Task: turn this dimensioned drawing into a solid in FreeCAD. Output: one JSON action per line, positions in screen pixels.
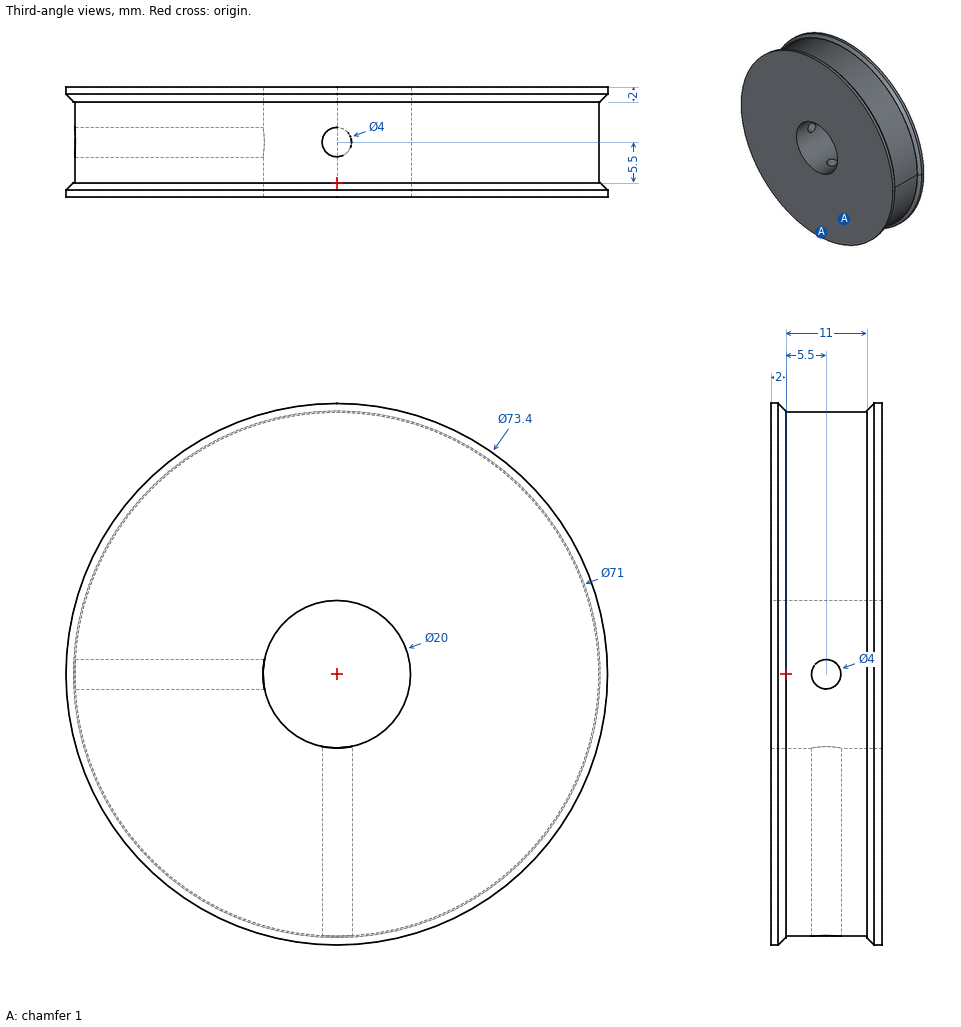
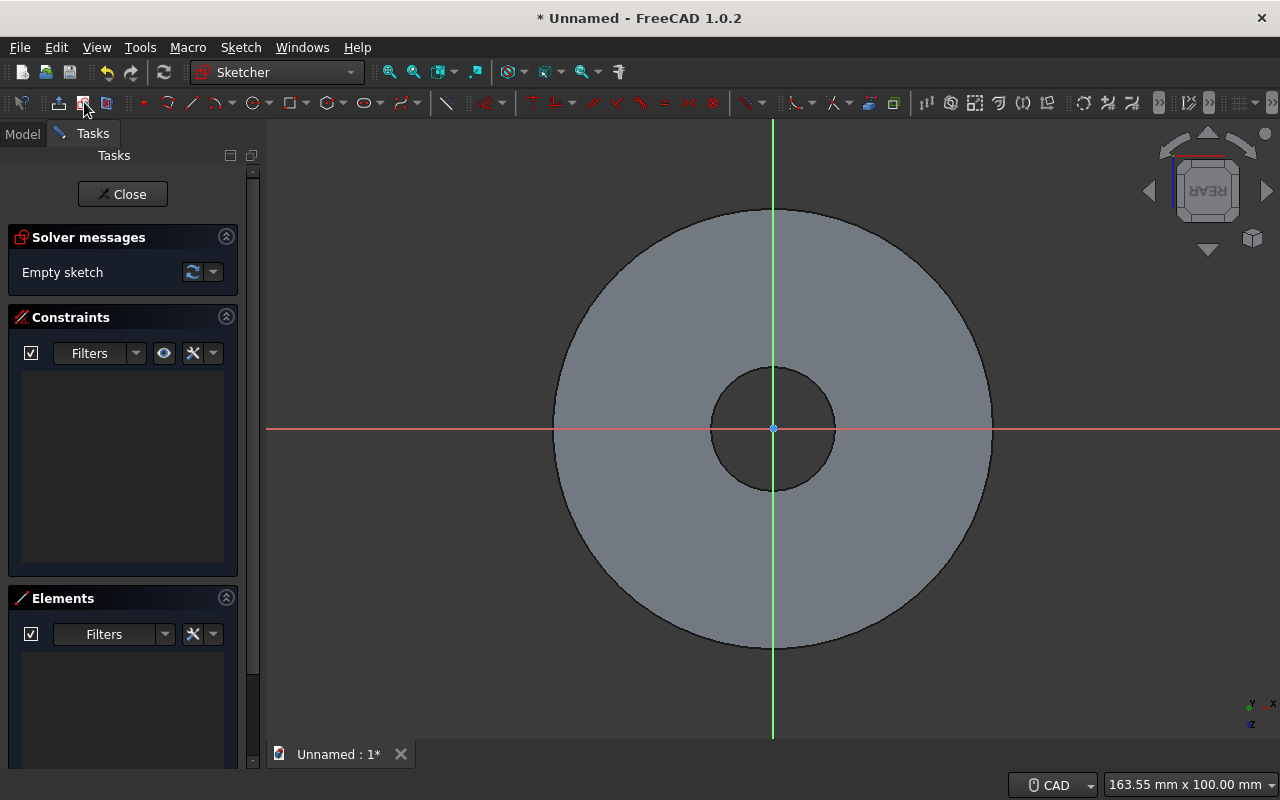
{"action": "left_click", "coordinate": [254, 104]}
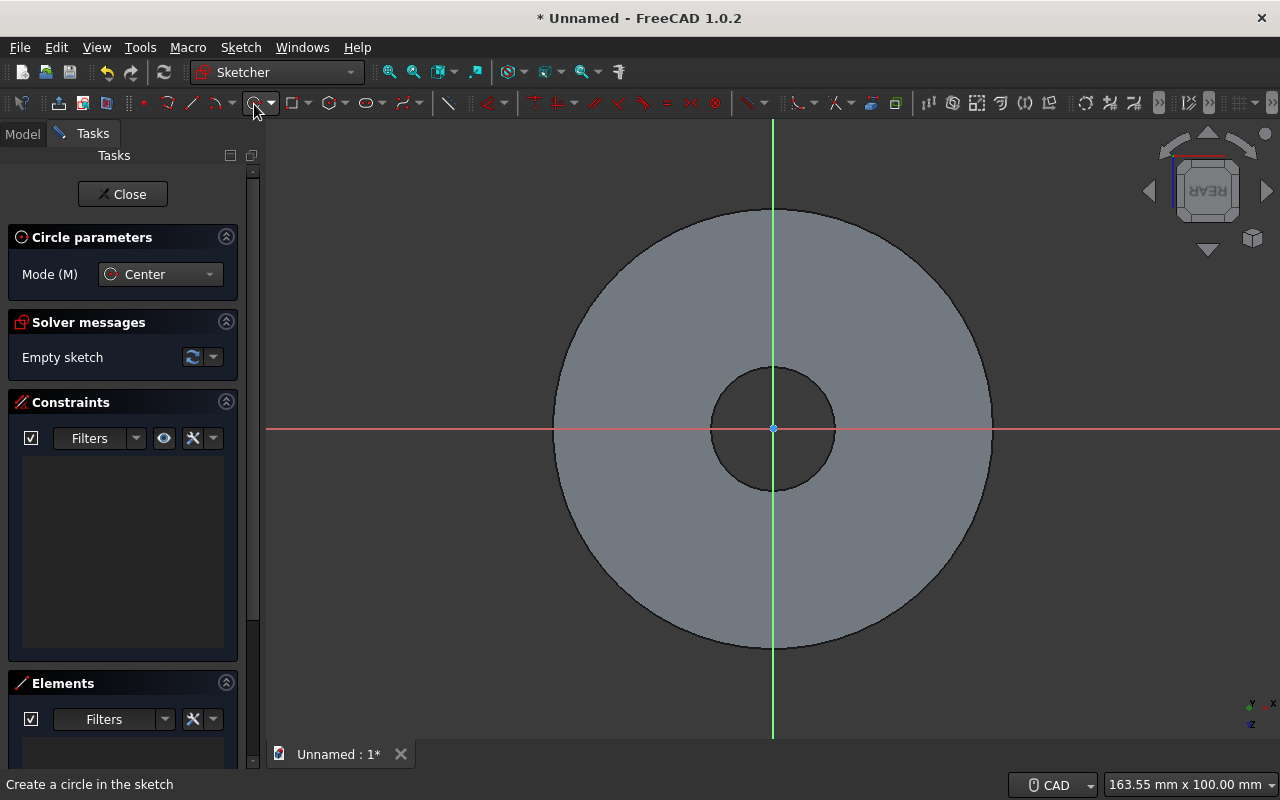
{"action": "left_click", "coordinate": [773, 429]}
{"action": "left_click", "coordinate": [934, 268]}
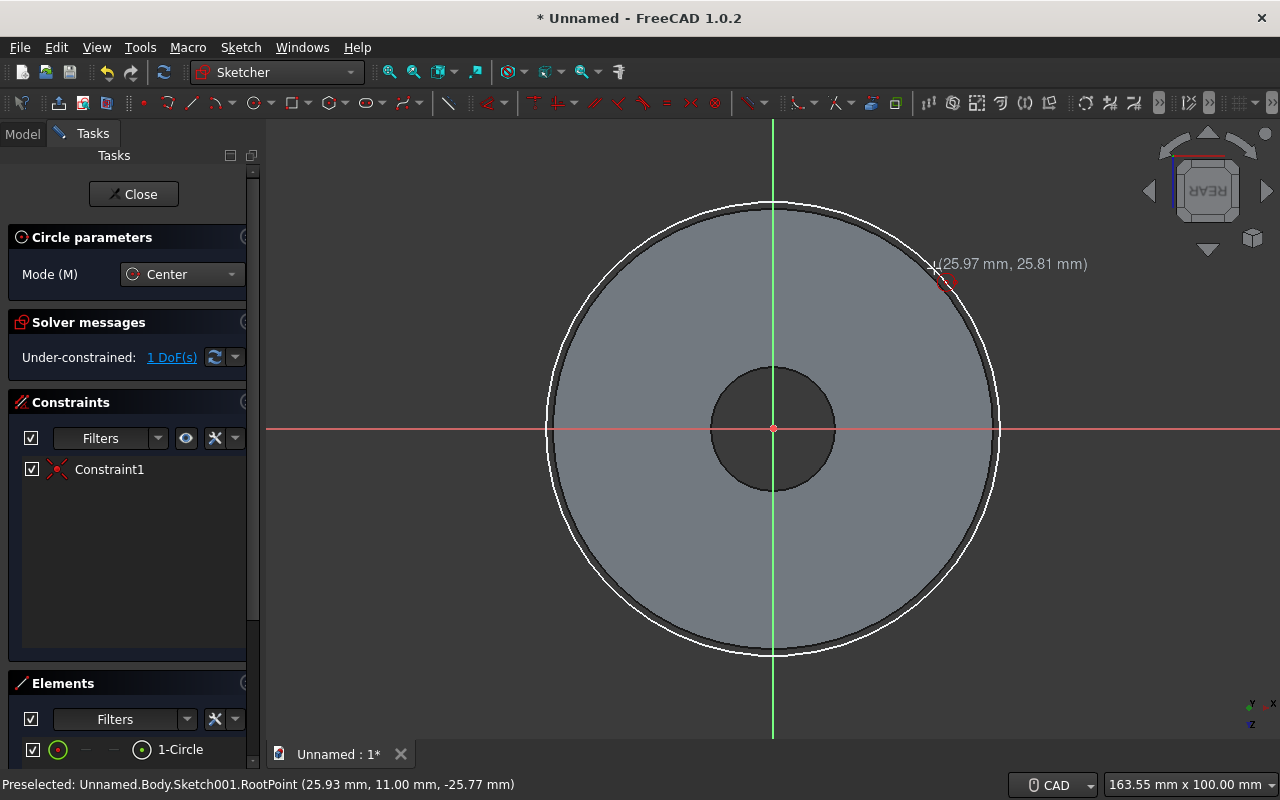
{"action": "left_click", "coordinate": [773, 429]}
{"action": "left_click", "coordinate": [817, 385]}
{"action": "key", "text": "Escape"}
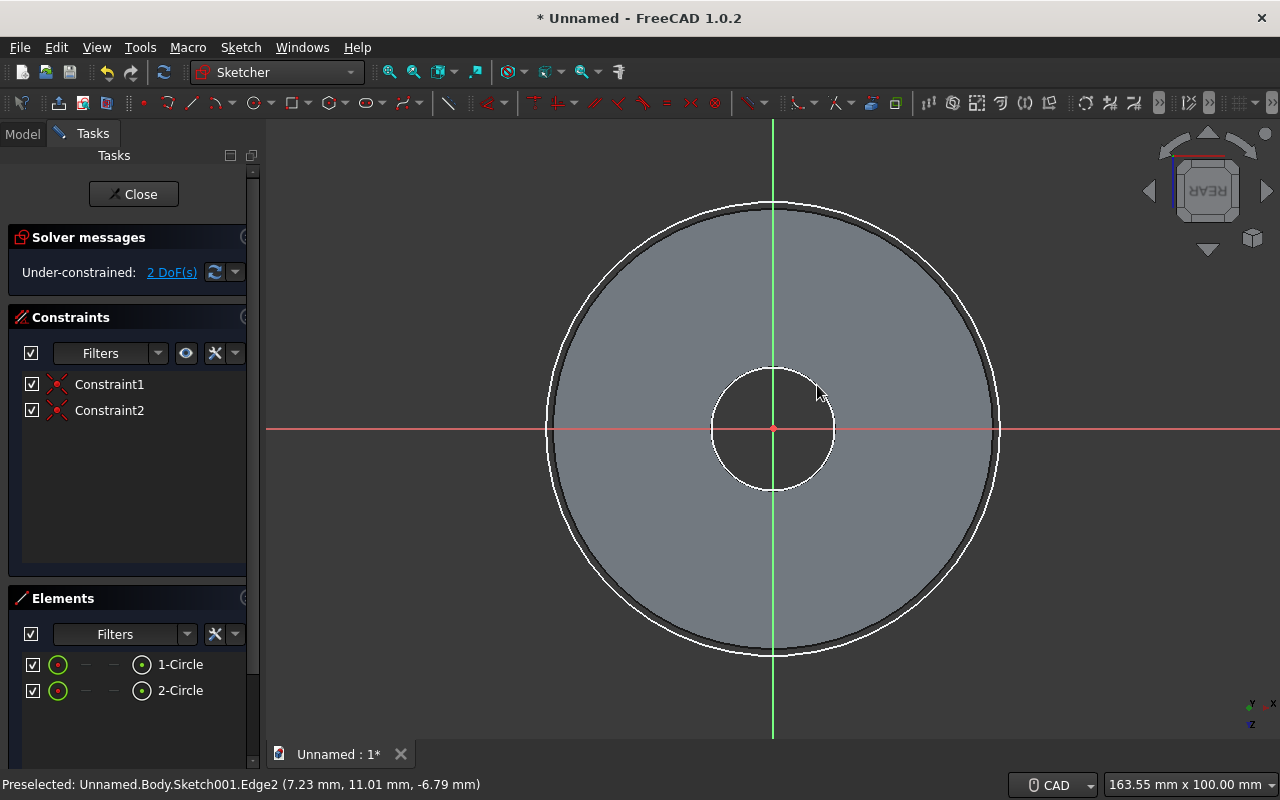
{"action": "left_click", "coordinate": [488, 104]}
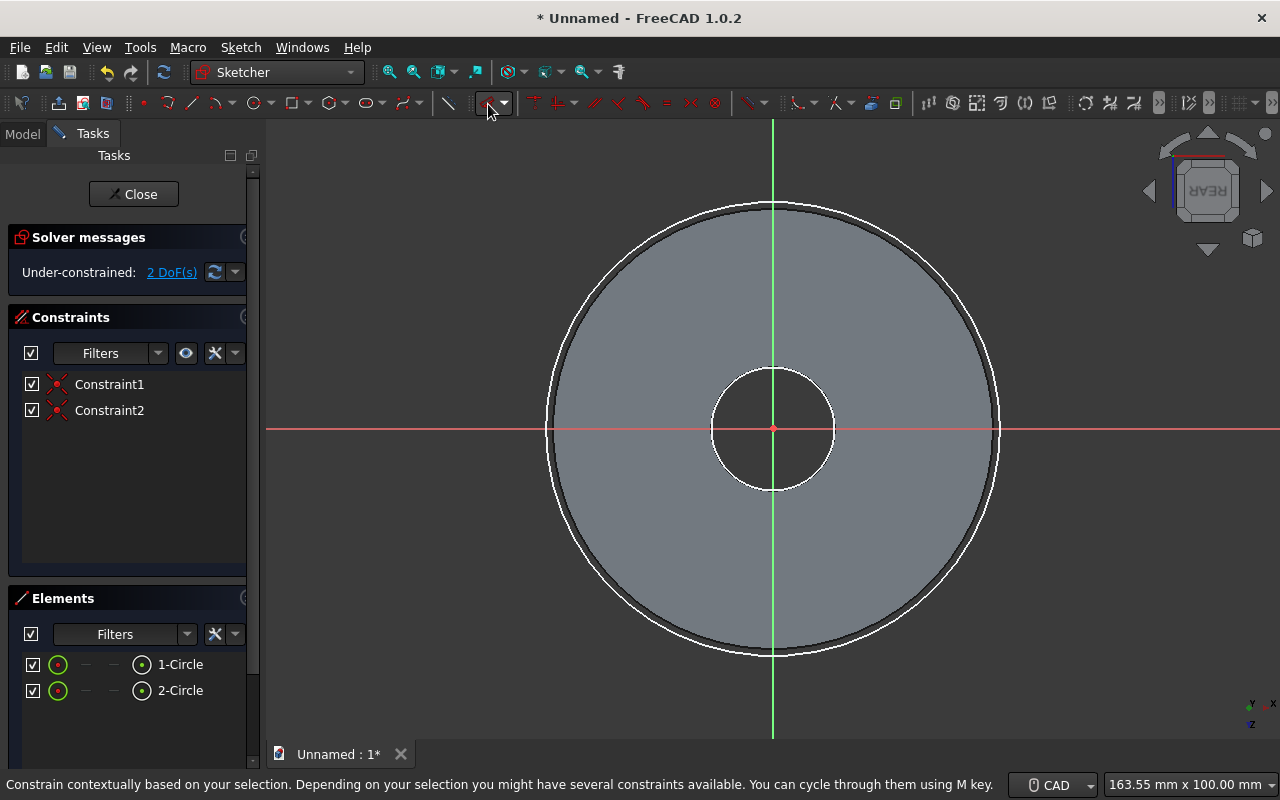
{"action": "left_click", "coordinate": [933, 268]}
{"action": "left_click", "coordinate": [956, 245]}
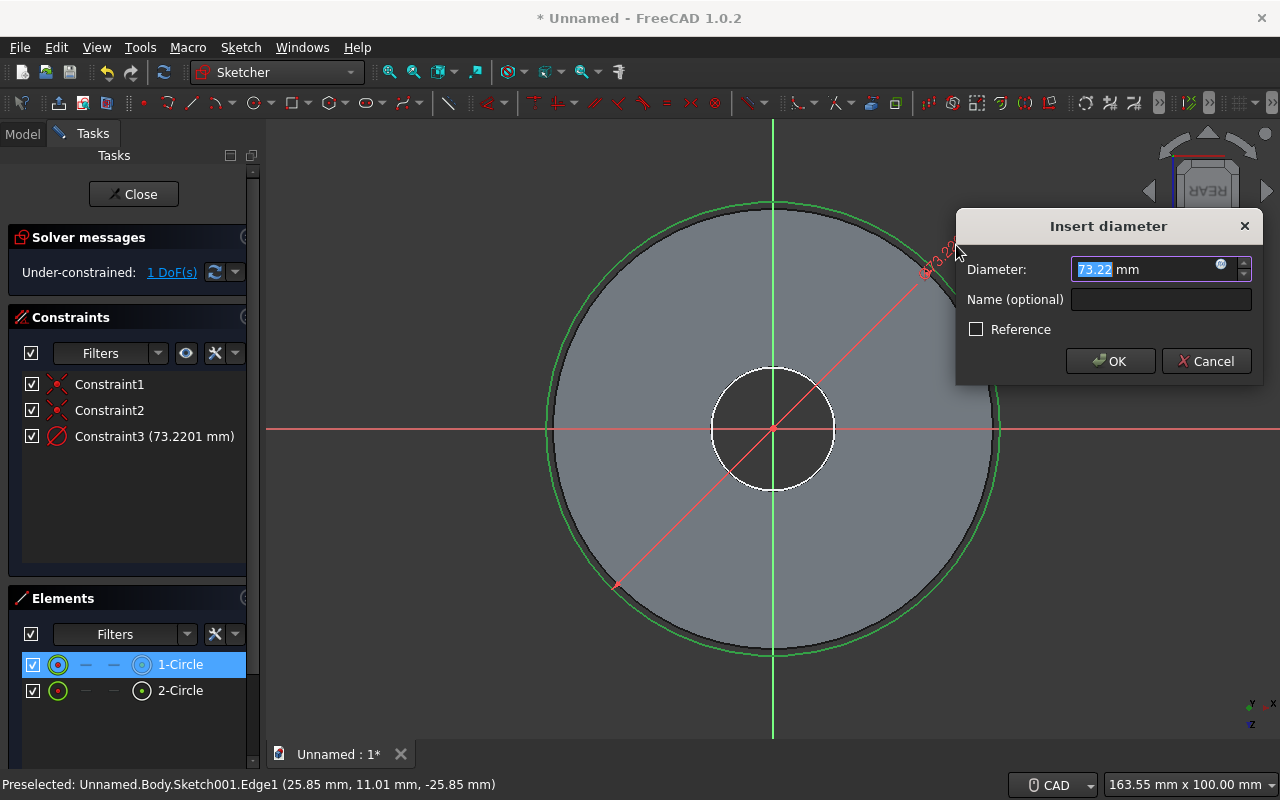
{"action": "type", "text": "73.4"}
{"action": "key", "text": "Return"}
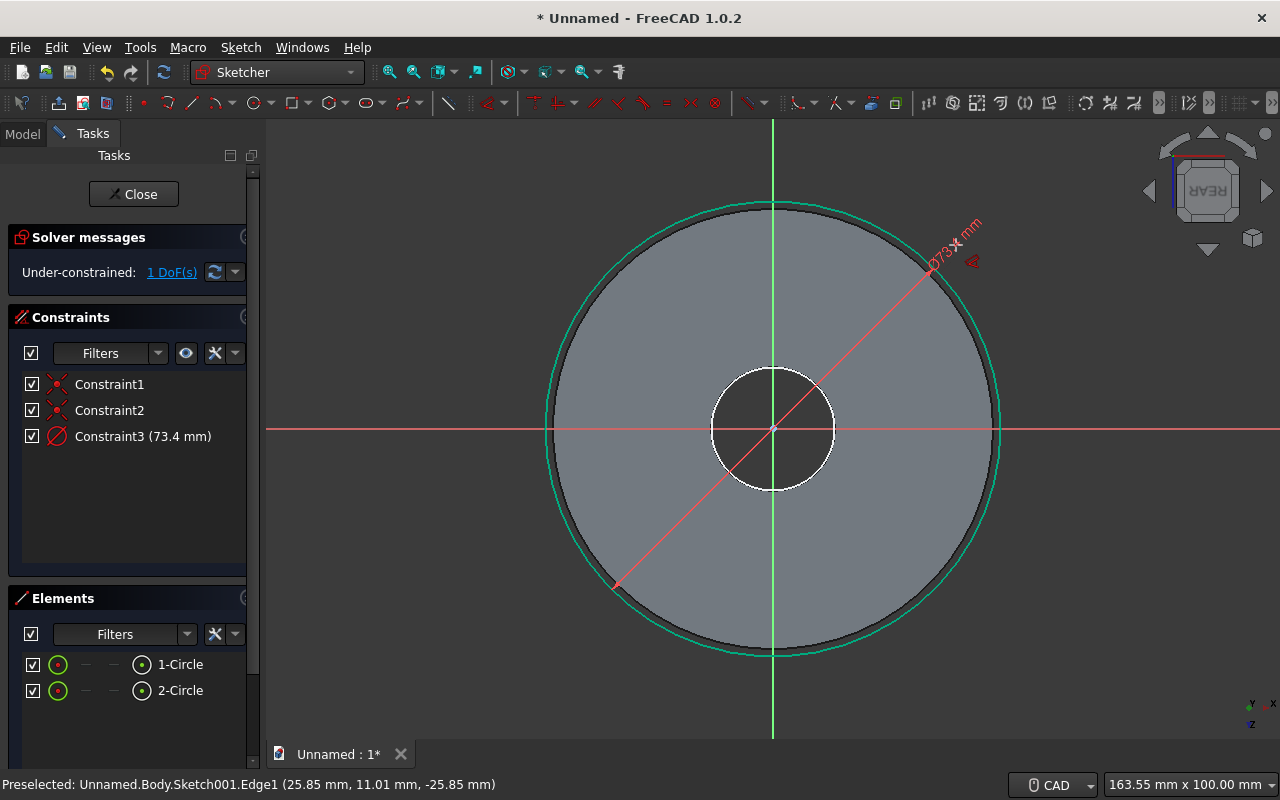
{"action": "left_click", "coordinate": [816, 385]}
{"action": "left_click", "coordinate": [838, 362]}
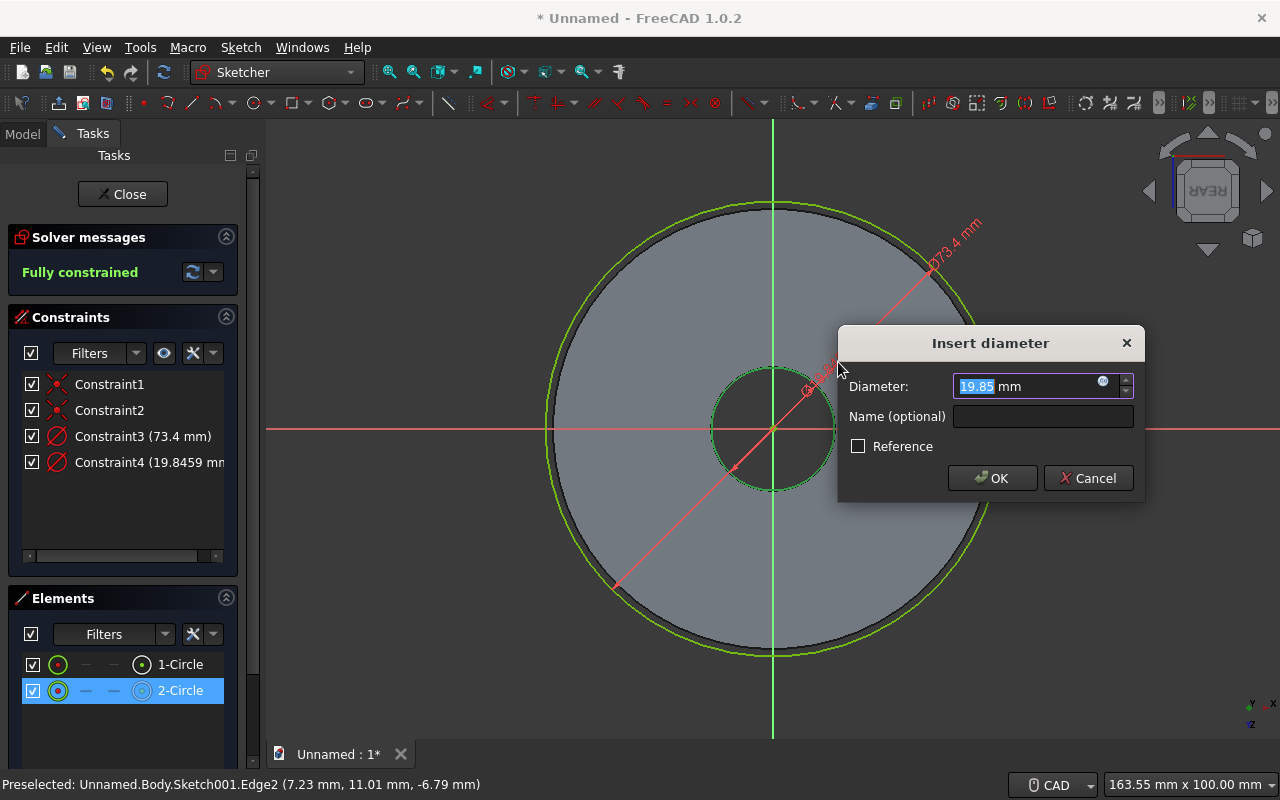
{"action": "type", "text": "20"}
{"action": "key", "text": "Return"}
{"action": "key", "text": "Escape"}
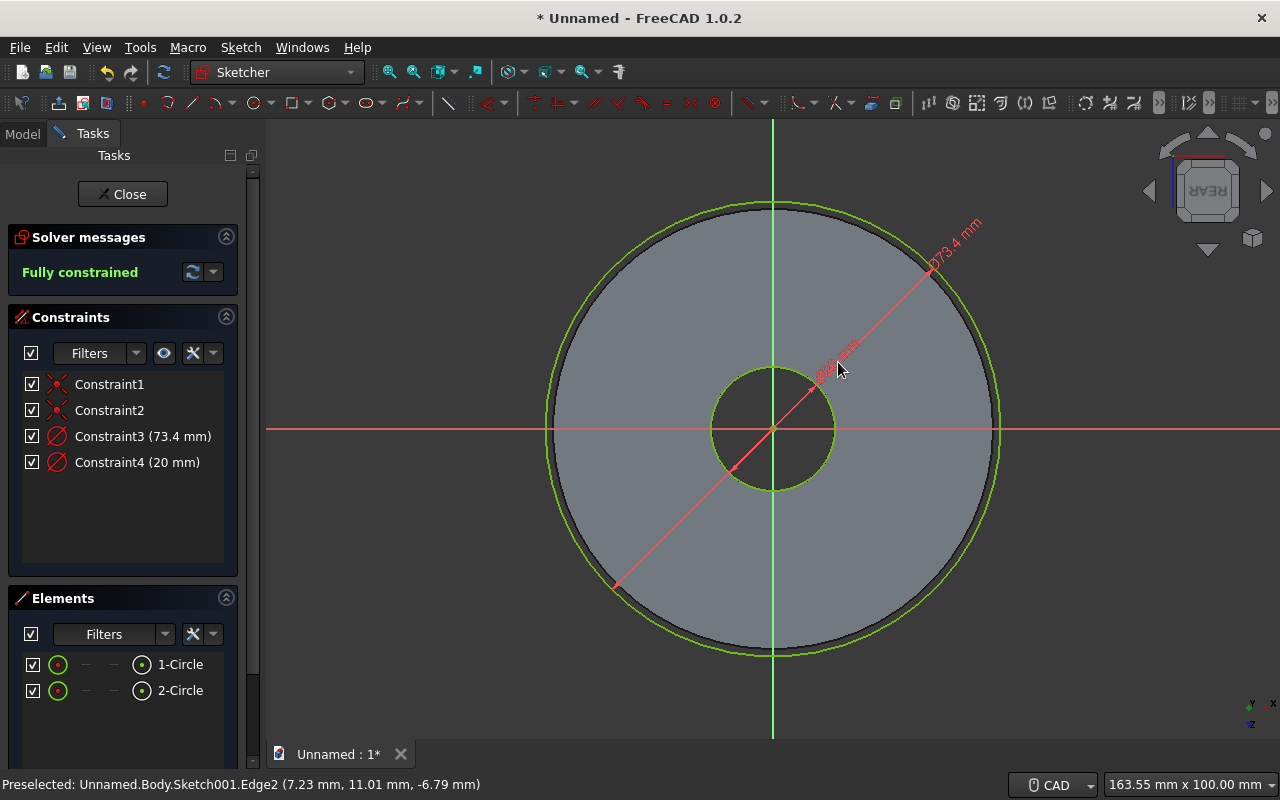
{"action": "left_click", "coordinate": [123, 194]}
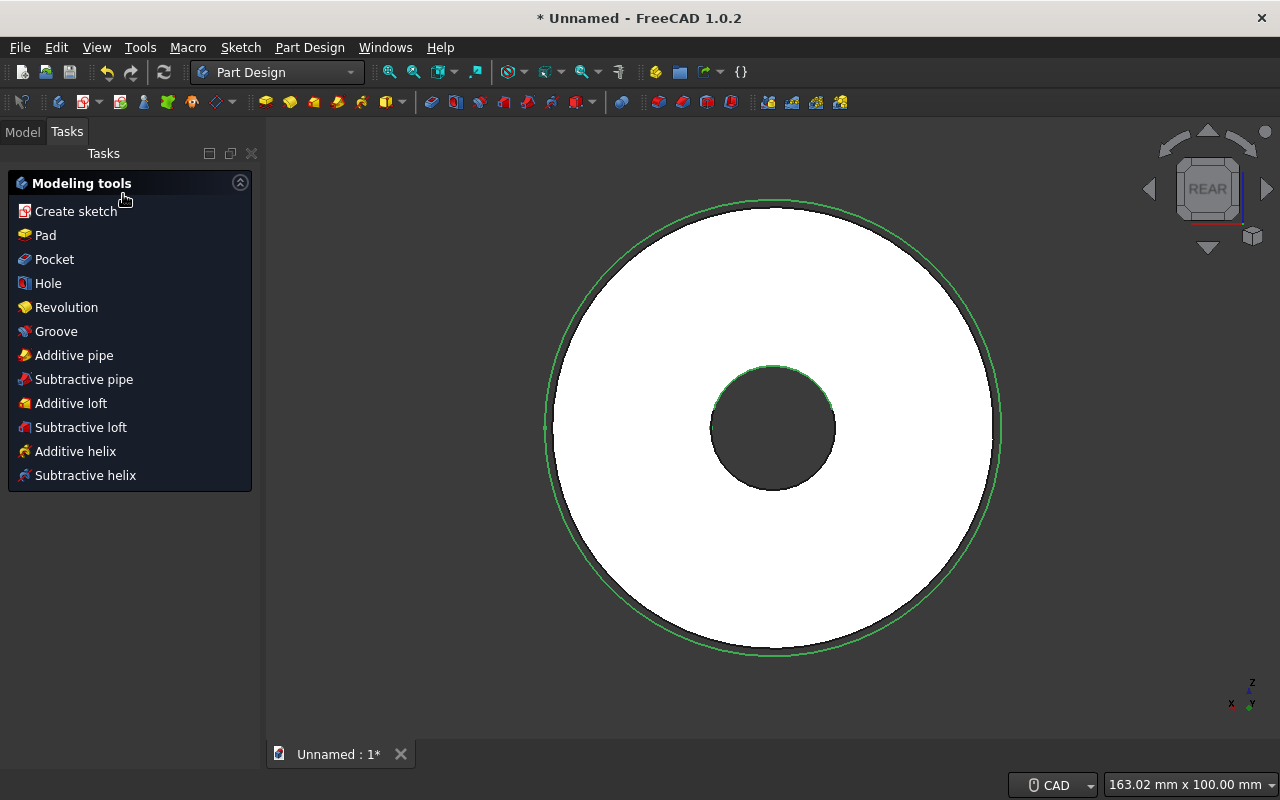
{"action": "left_click", "coordinate": [266, 102]}